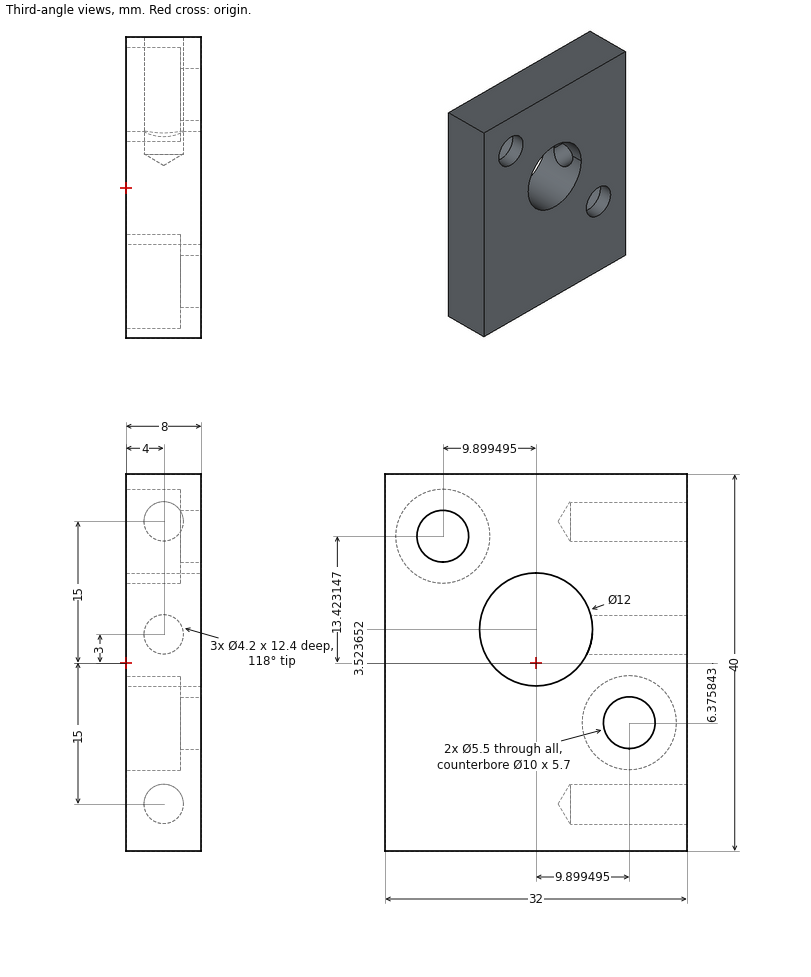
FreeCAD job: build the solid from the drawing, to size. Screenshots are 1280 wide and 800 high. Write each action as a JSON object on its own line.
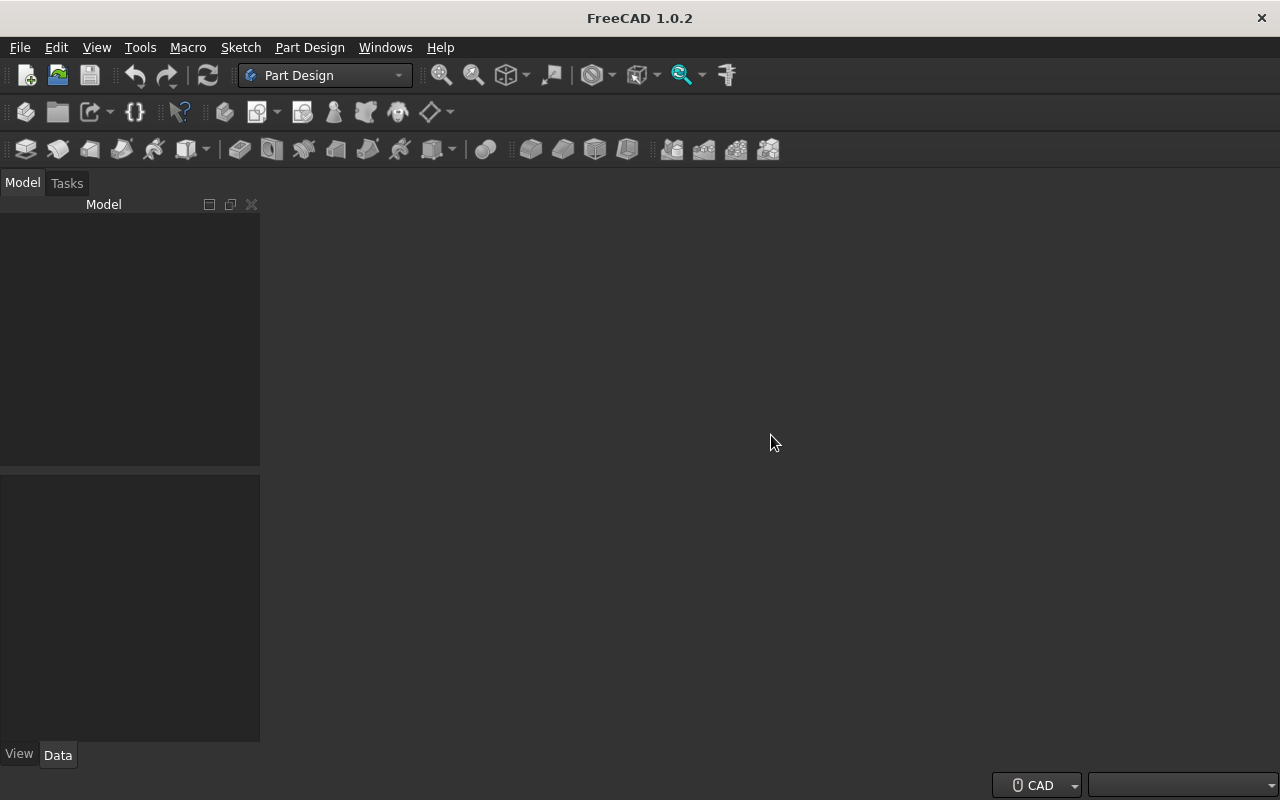
{"action": "left_click", "coordinate": [26, 76]}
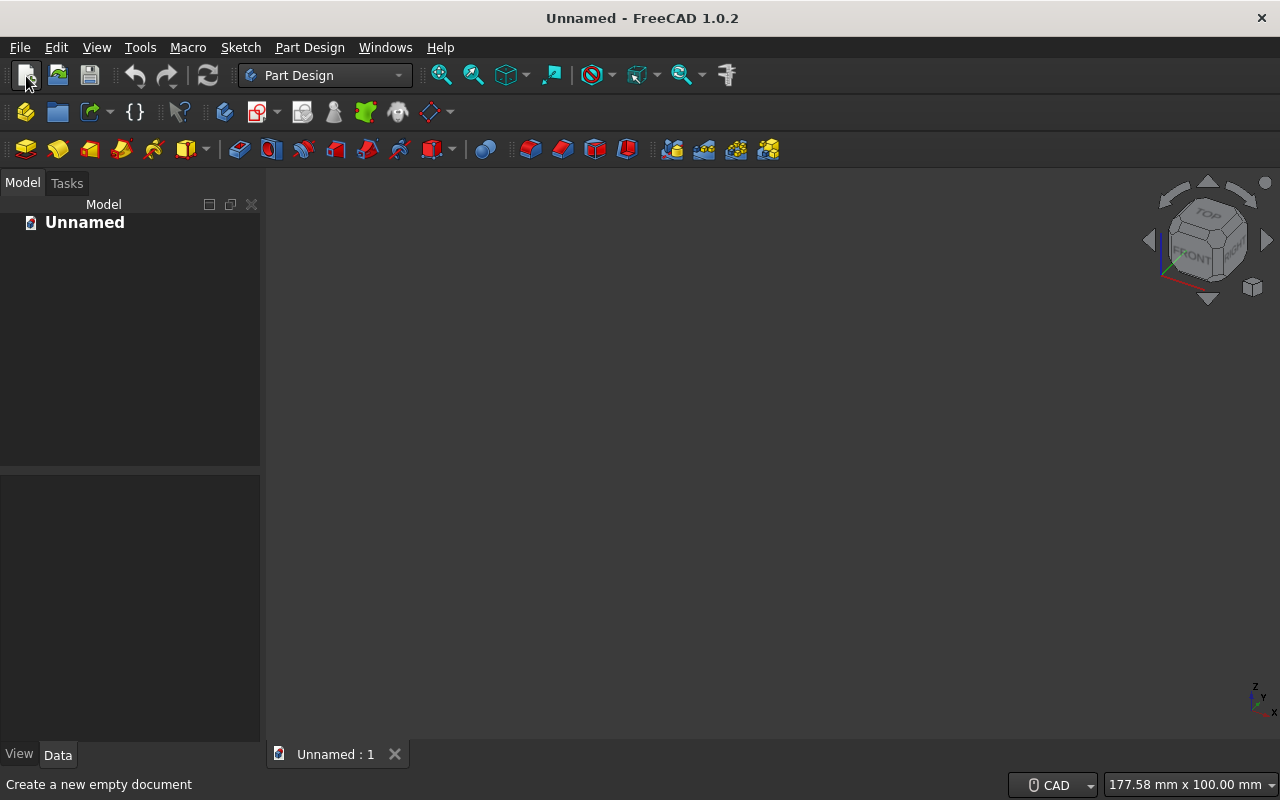
{"action": "left_click", "coordinate": [258, 112]}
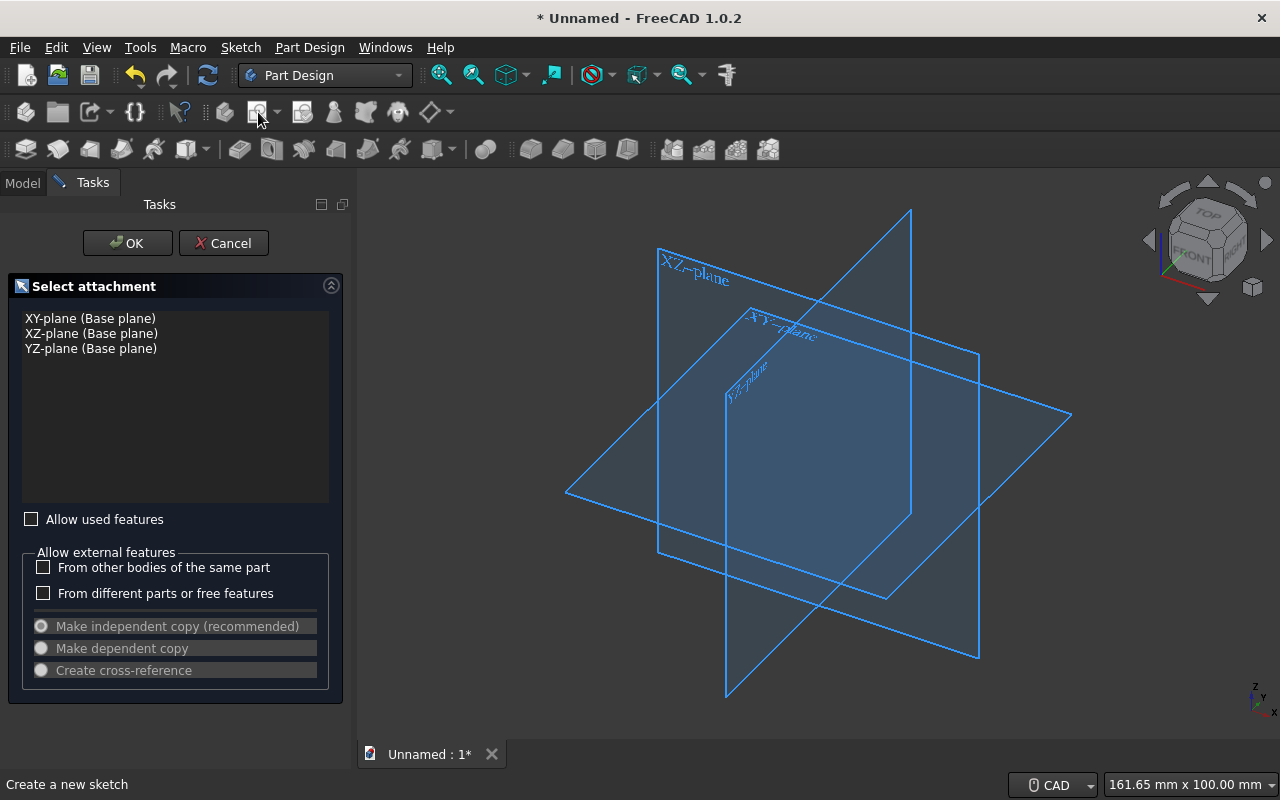
{"action": "left_click", "coordinate": [82, 348]}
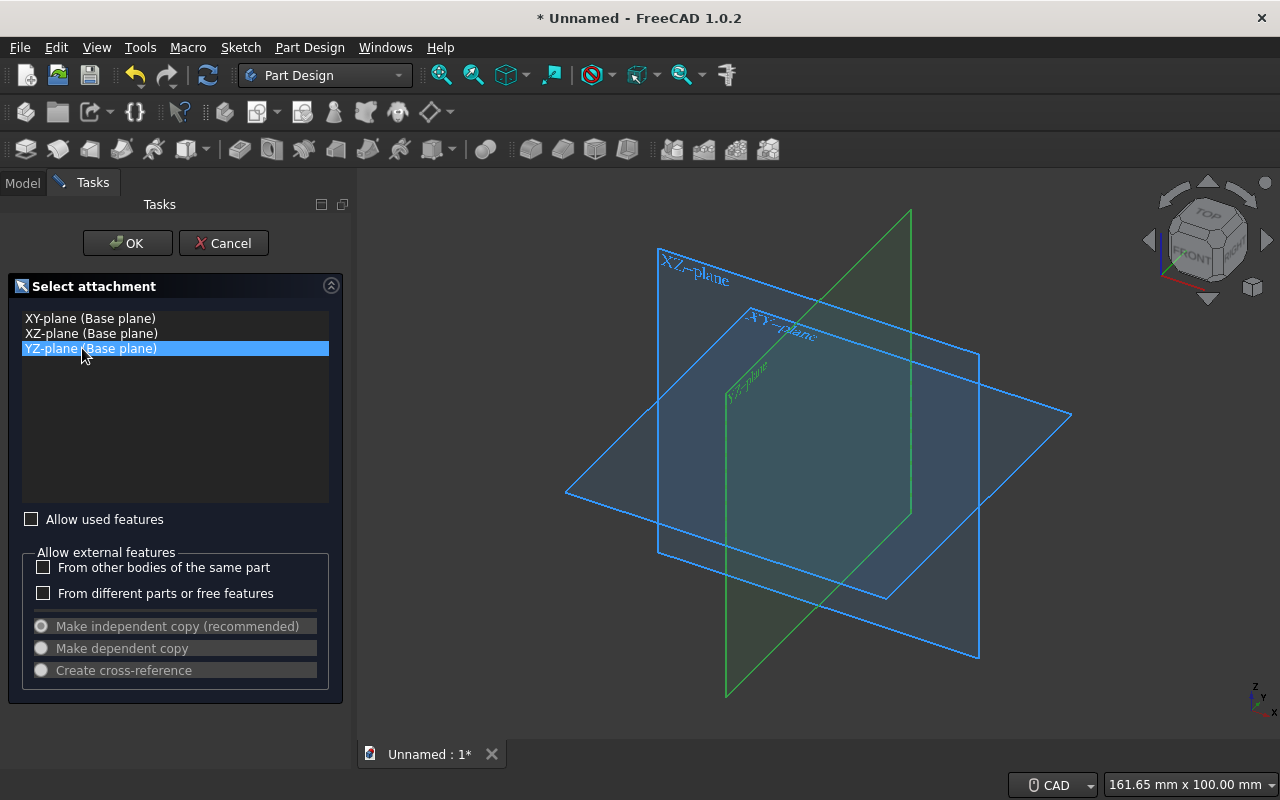
{"action": "left_click", "coordinate": [128, 243]}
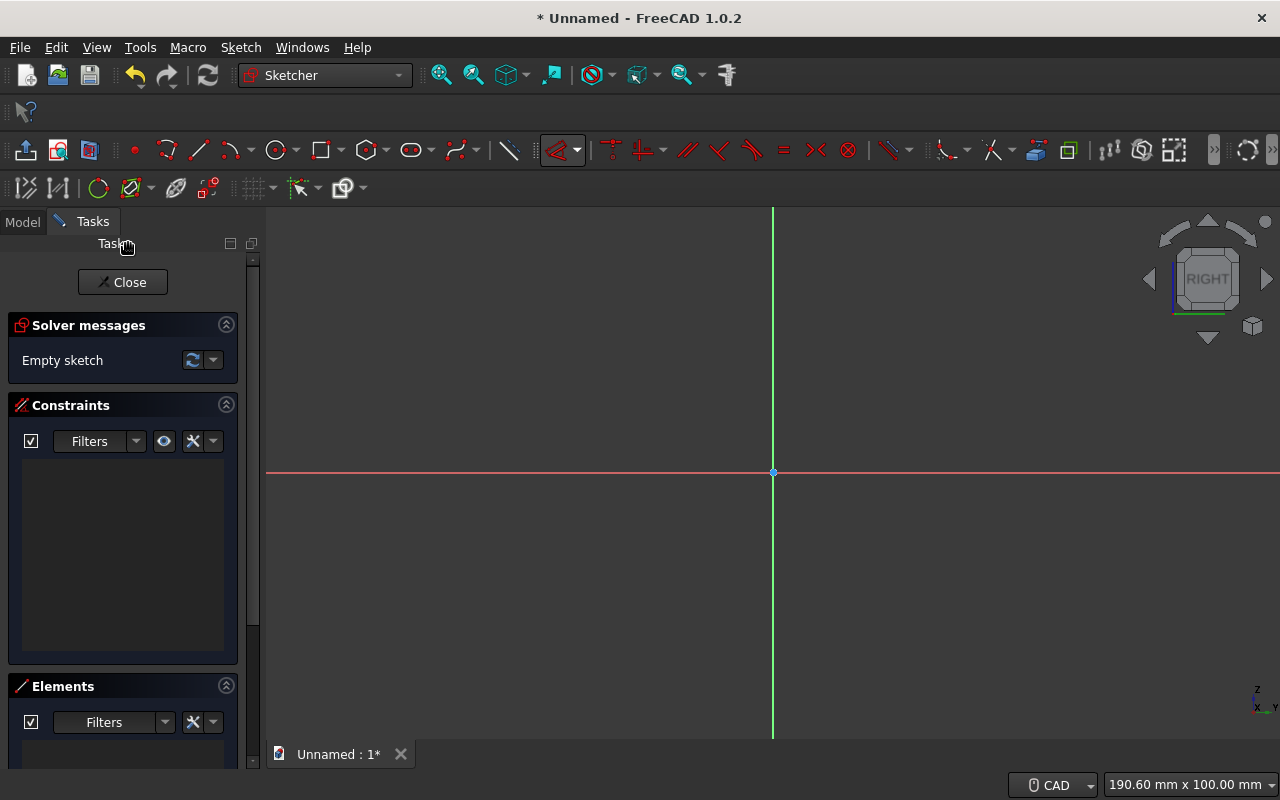
{"action": "scroll", "coordinate": [912, 473], "scroll_direction": "up", "scroll_amount": 2}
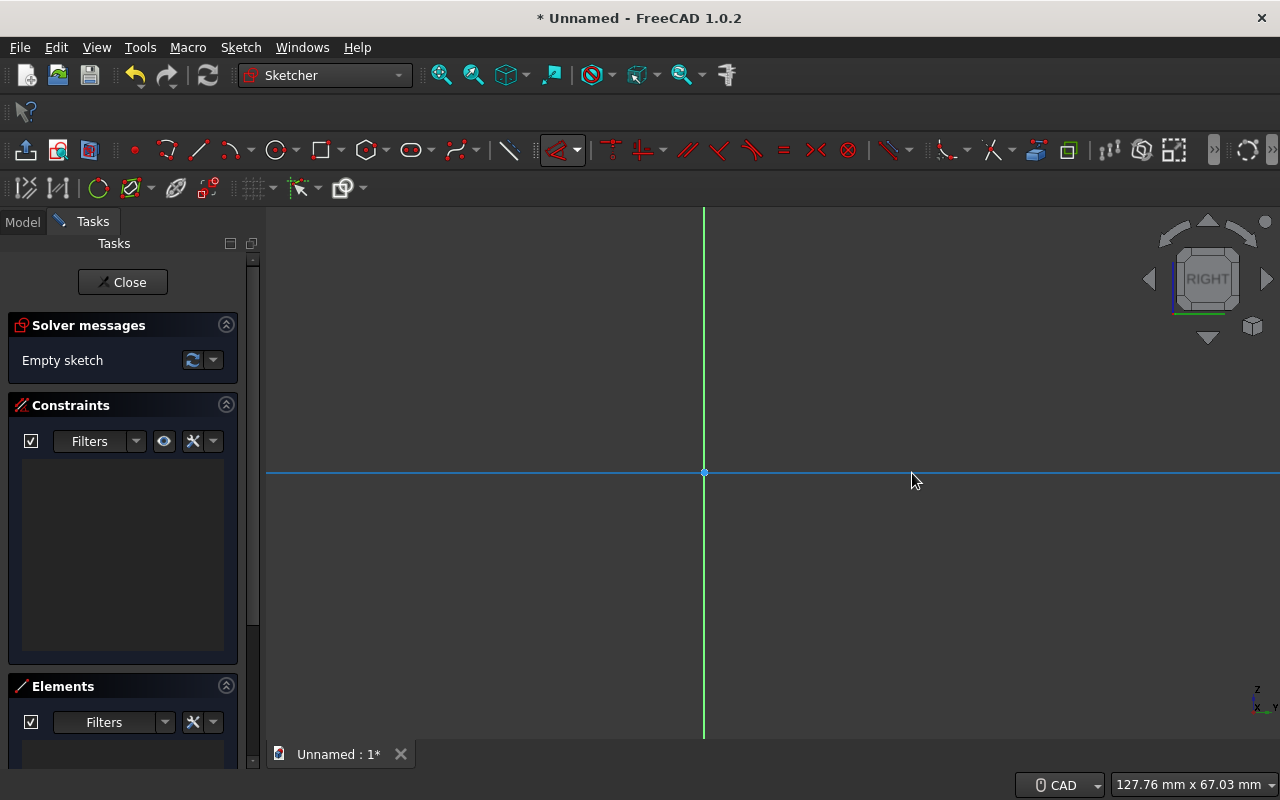
{"action": "key", "text": "g v"}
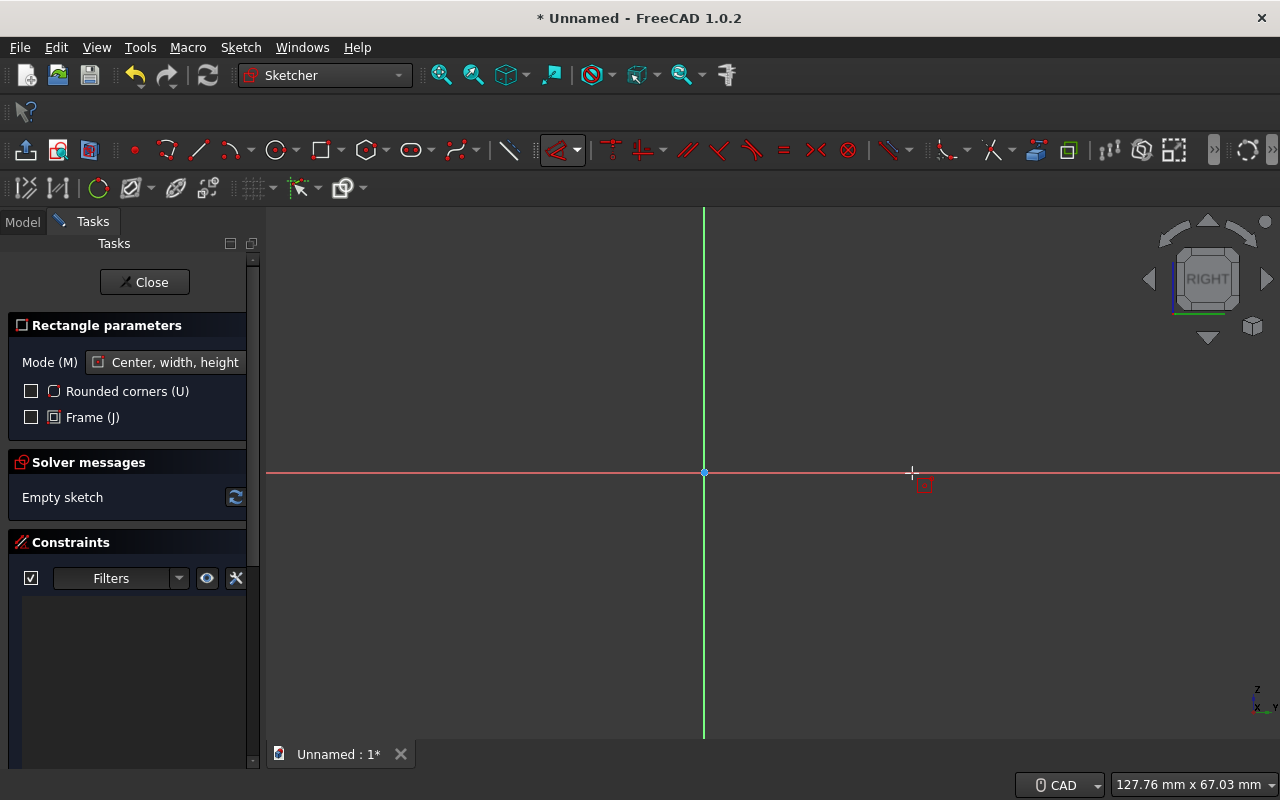
{"action": "left_click", "coordinate": [704, 473]}
{"action": "mouse_move", "coordinate": [831, 314]}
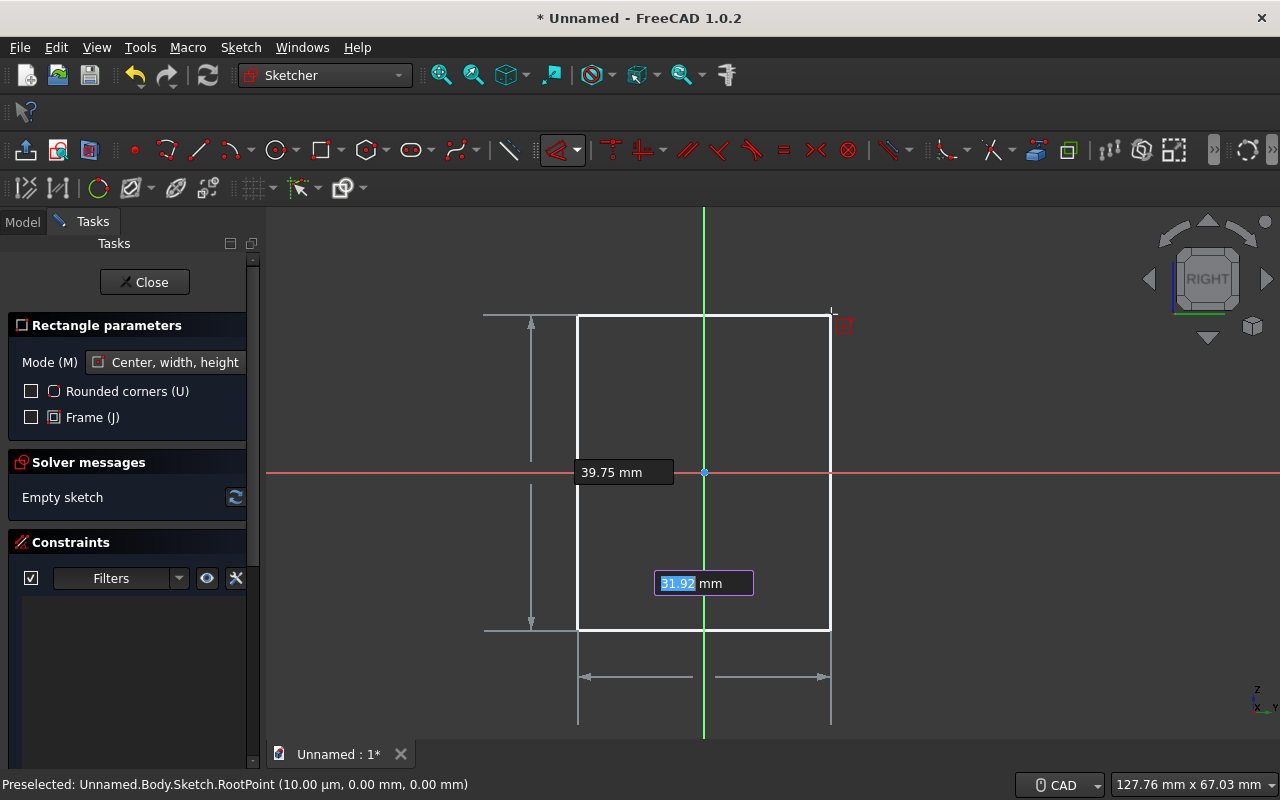
{"action": "type", "text": "32"}
{"action": "key", "text": "Tab"}
{"action": "type", "text": "40"}
{"action": "key", "text": "Return"}
{"action": "key", "text": "Escape"}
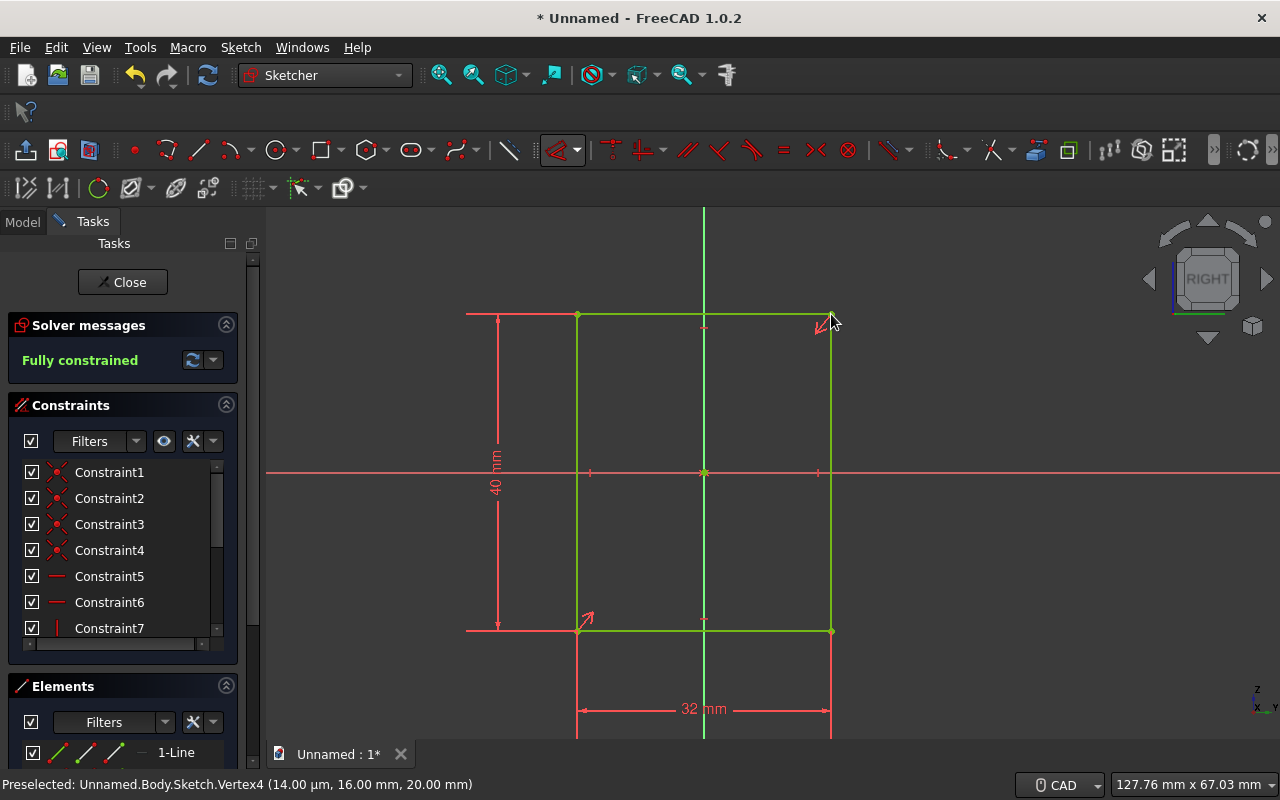
{"action": "left_click", "coordinate": [123, 282]}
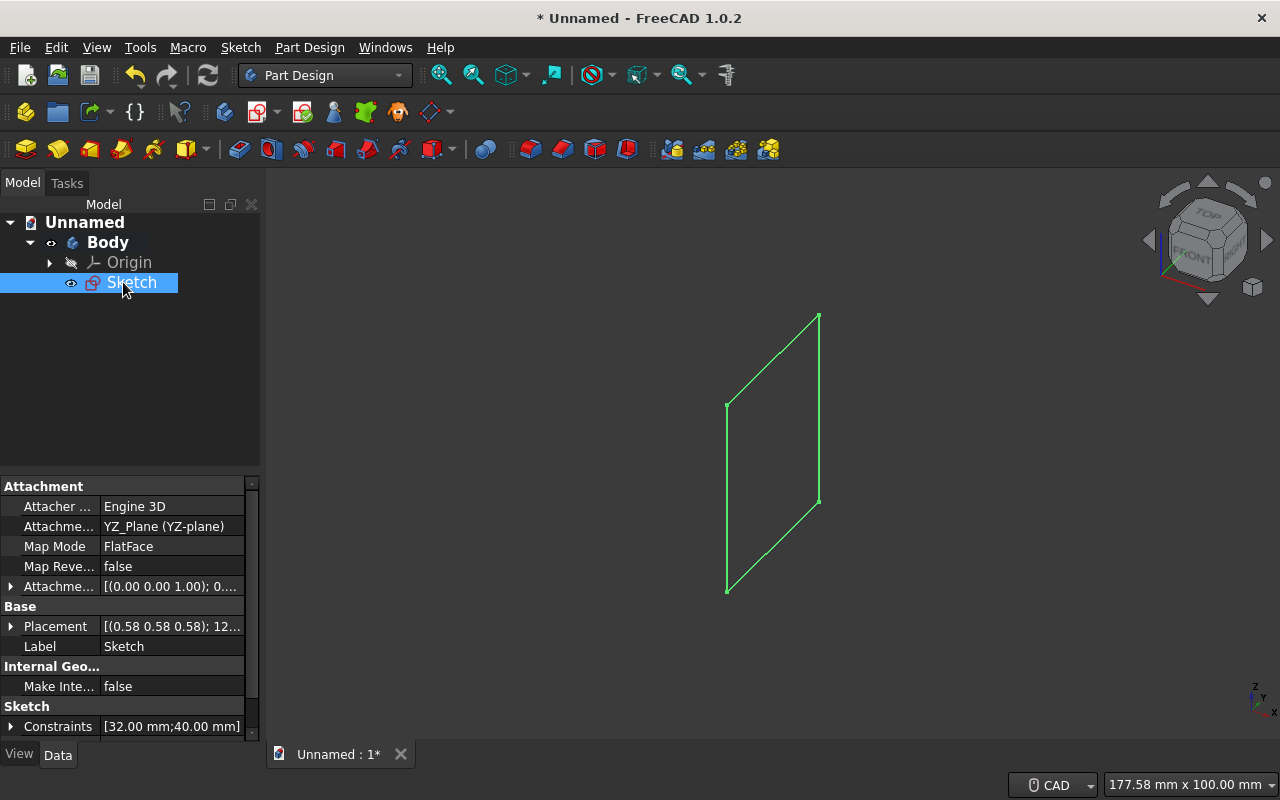
{"action": "left_click", "coordinate": [26, 150]}